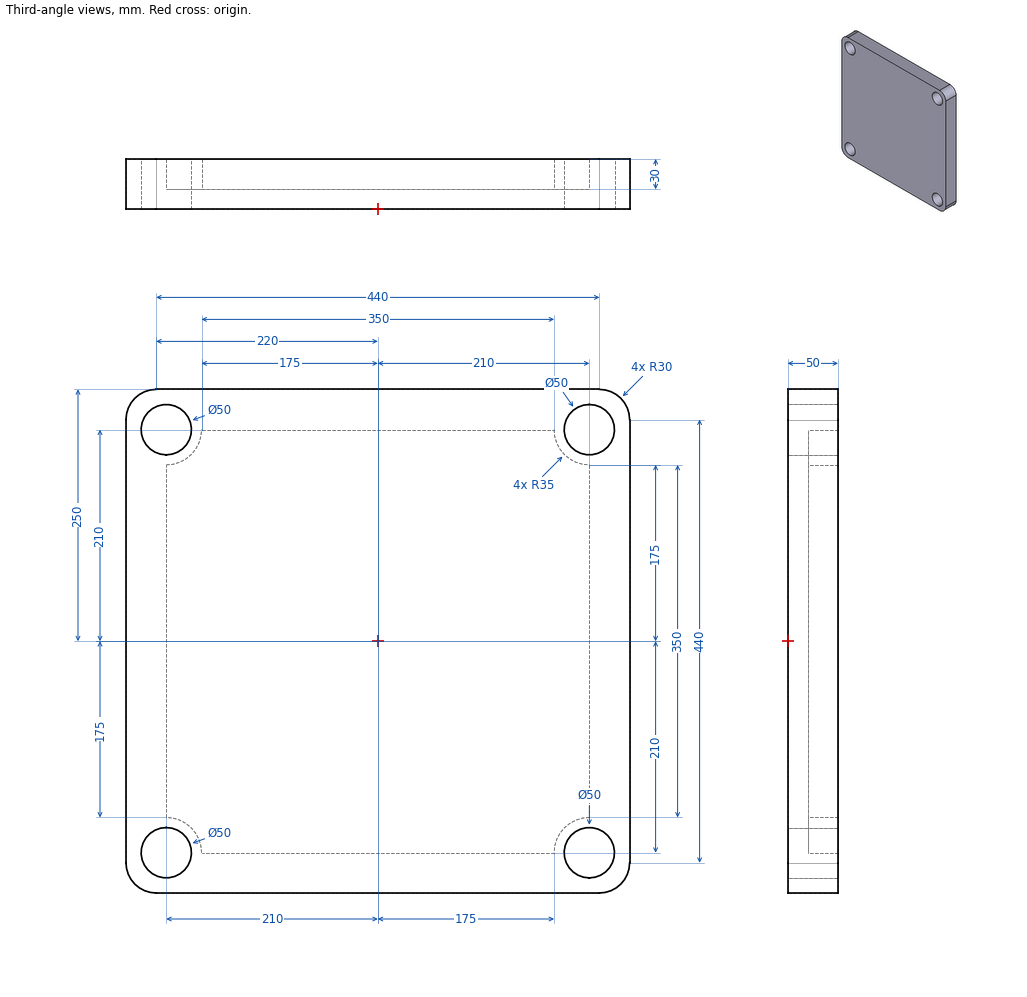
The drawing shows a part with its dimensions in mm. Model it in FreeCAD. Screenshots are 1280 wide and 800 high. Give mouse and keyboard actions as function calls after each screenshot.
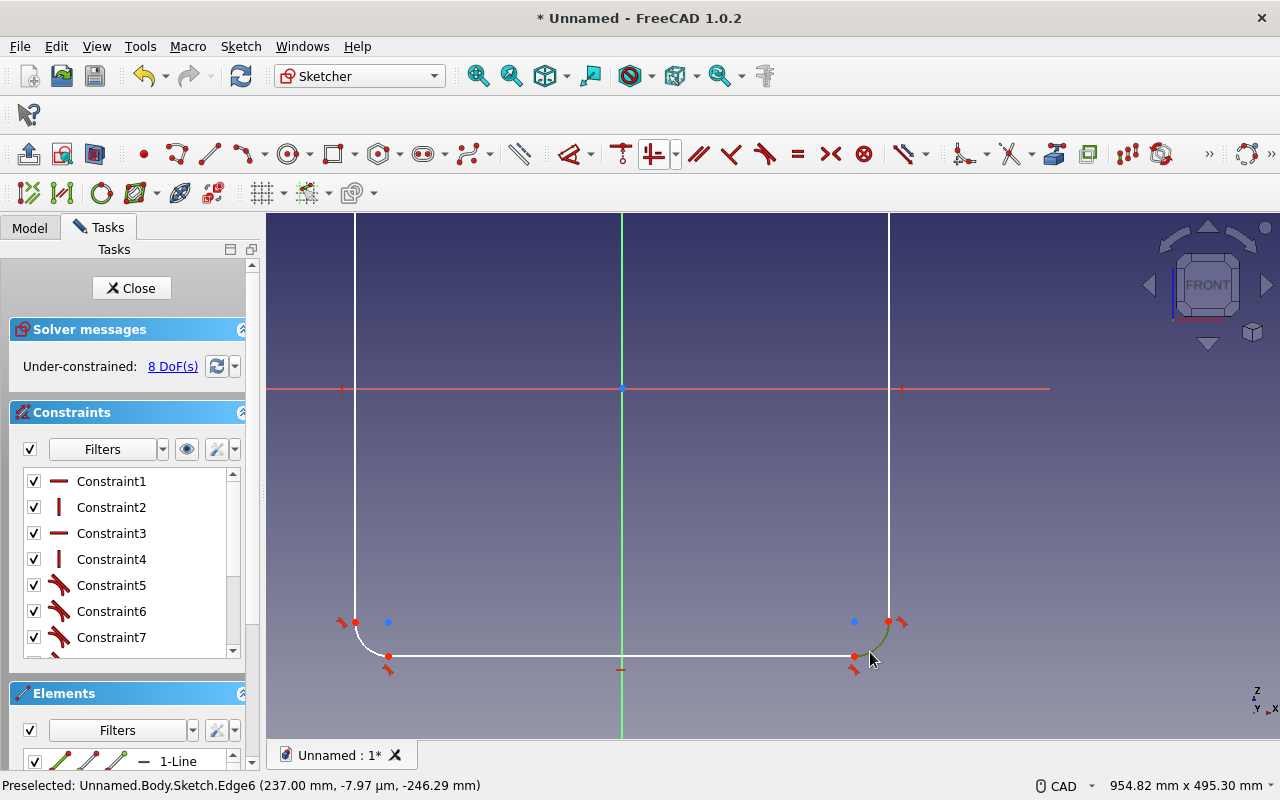
click(359, 638)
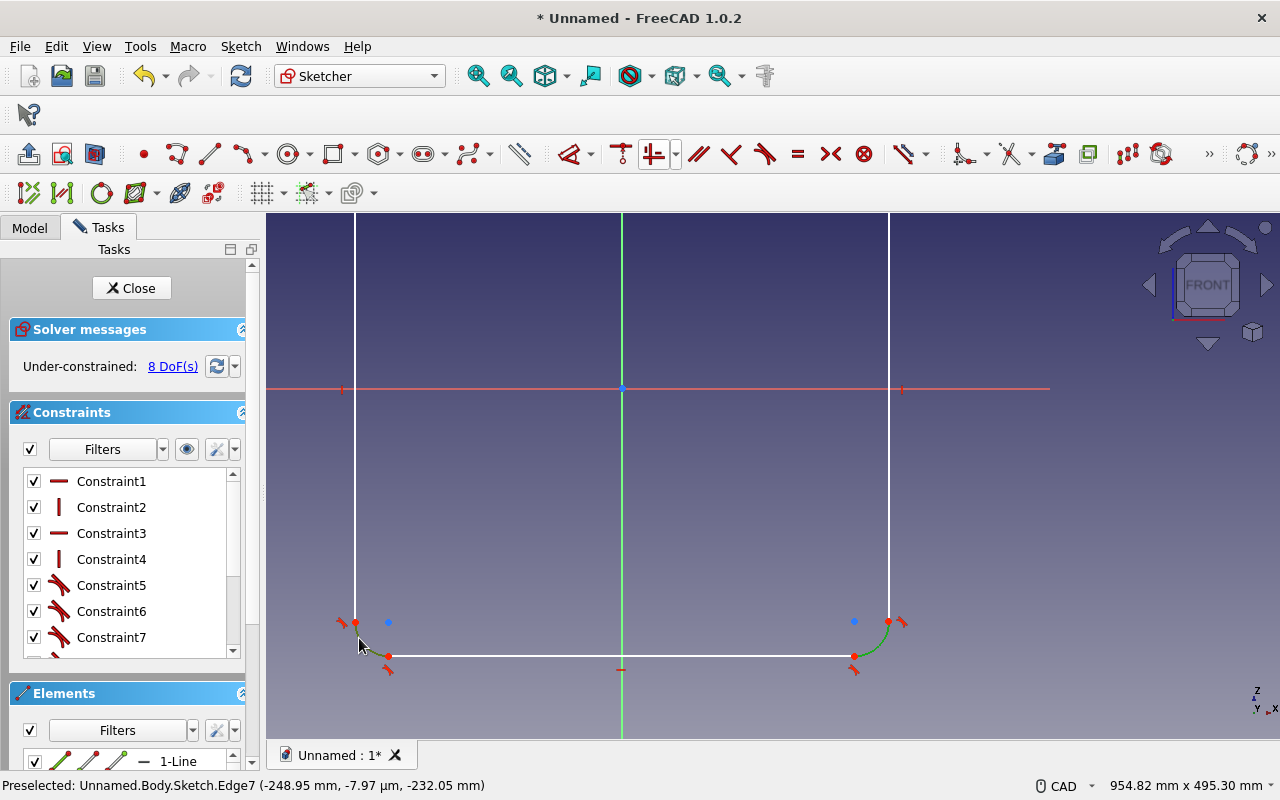
scroll(872, 653, down, 2)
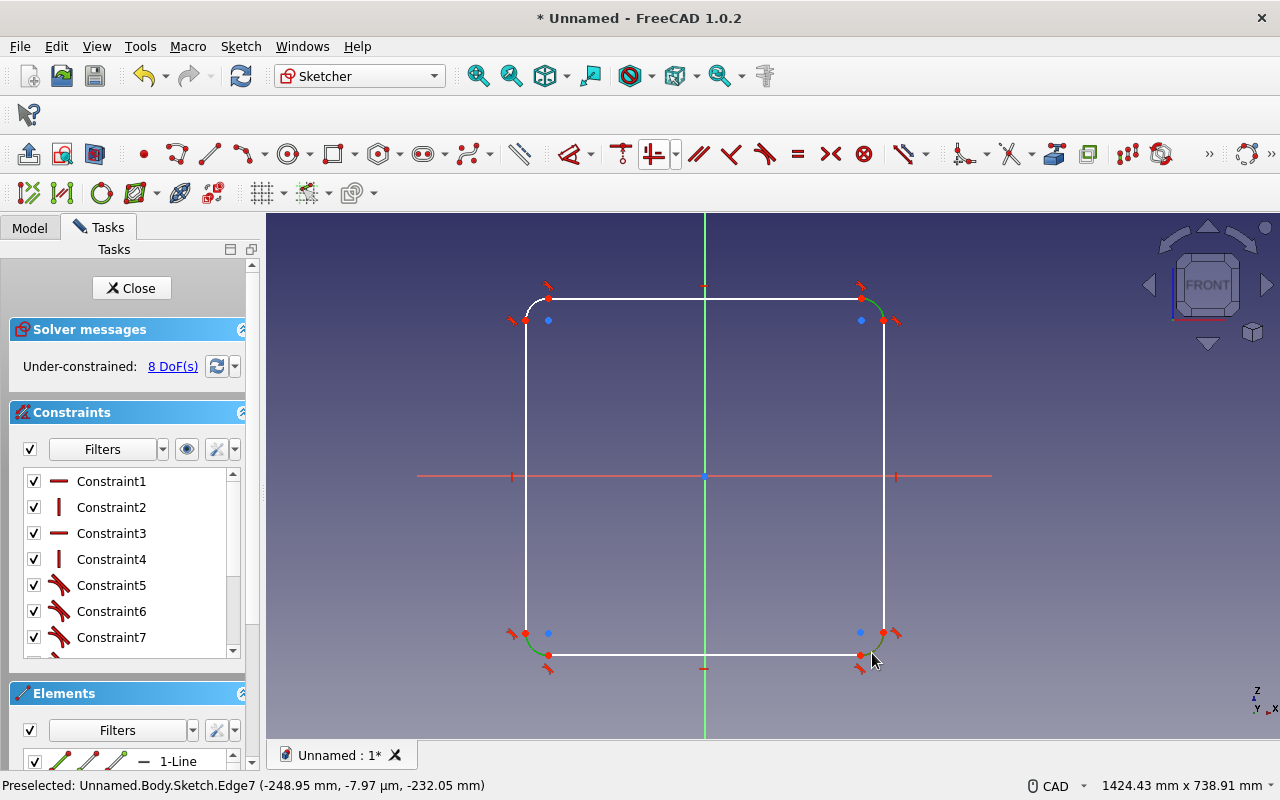
scroll(538, 301, up, 2)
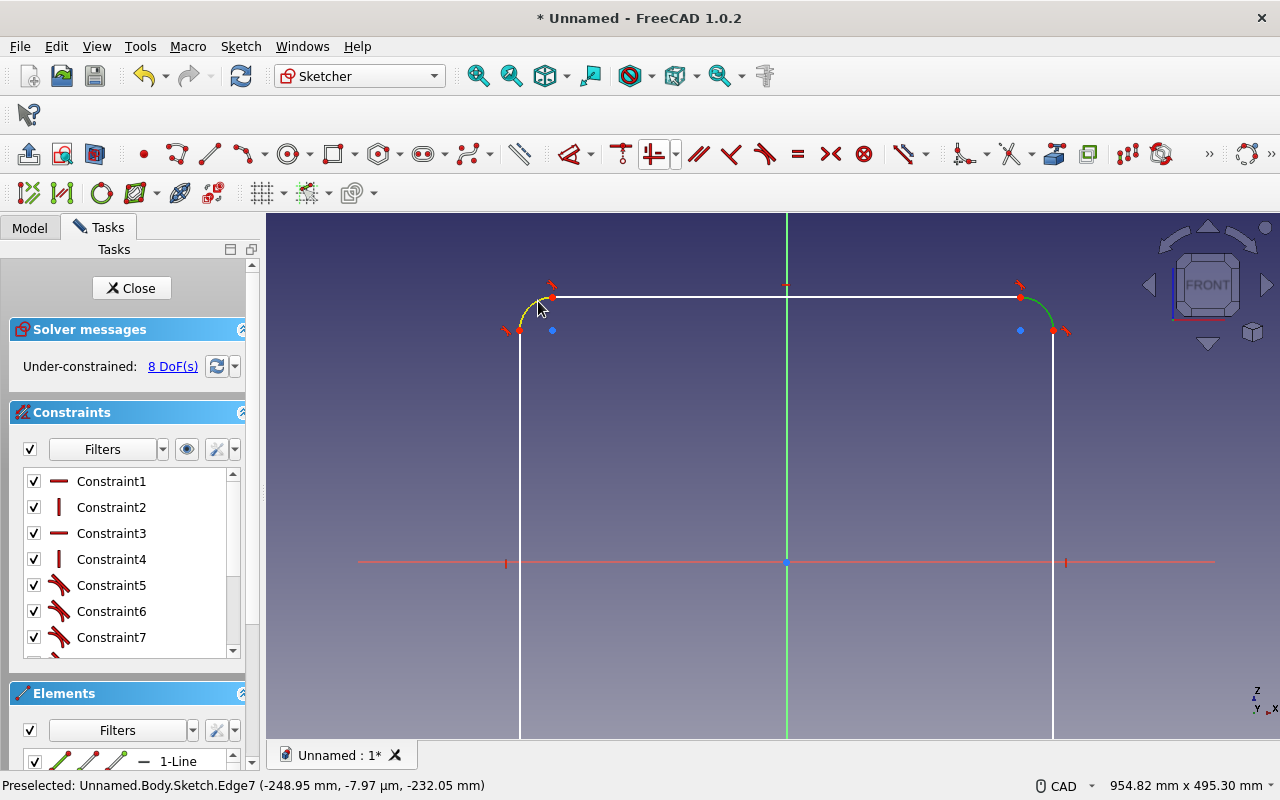
click(538, 301)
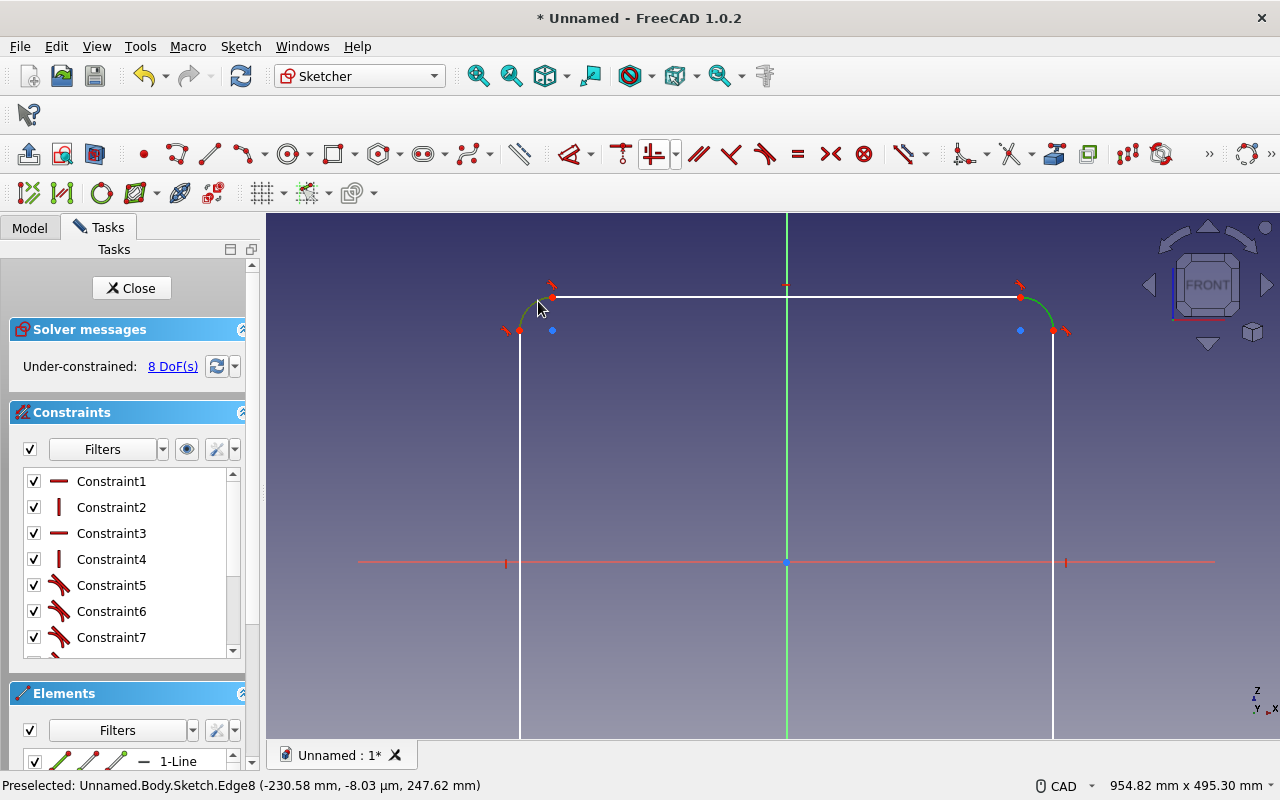
click(798, 154)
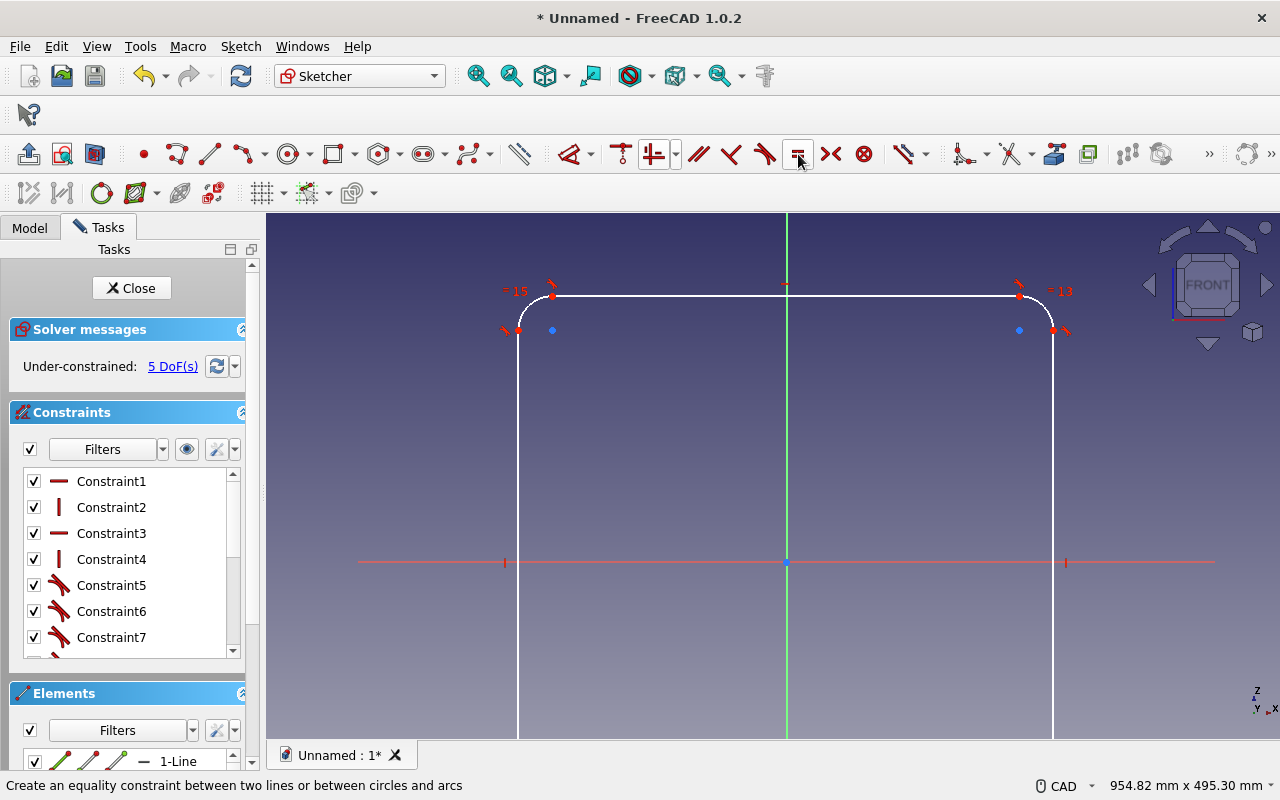
click(568, 154)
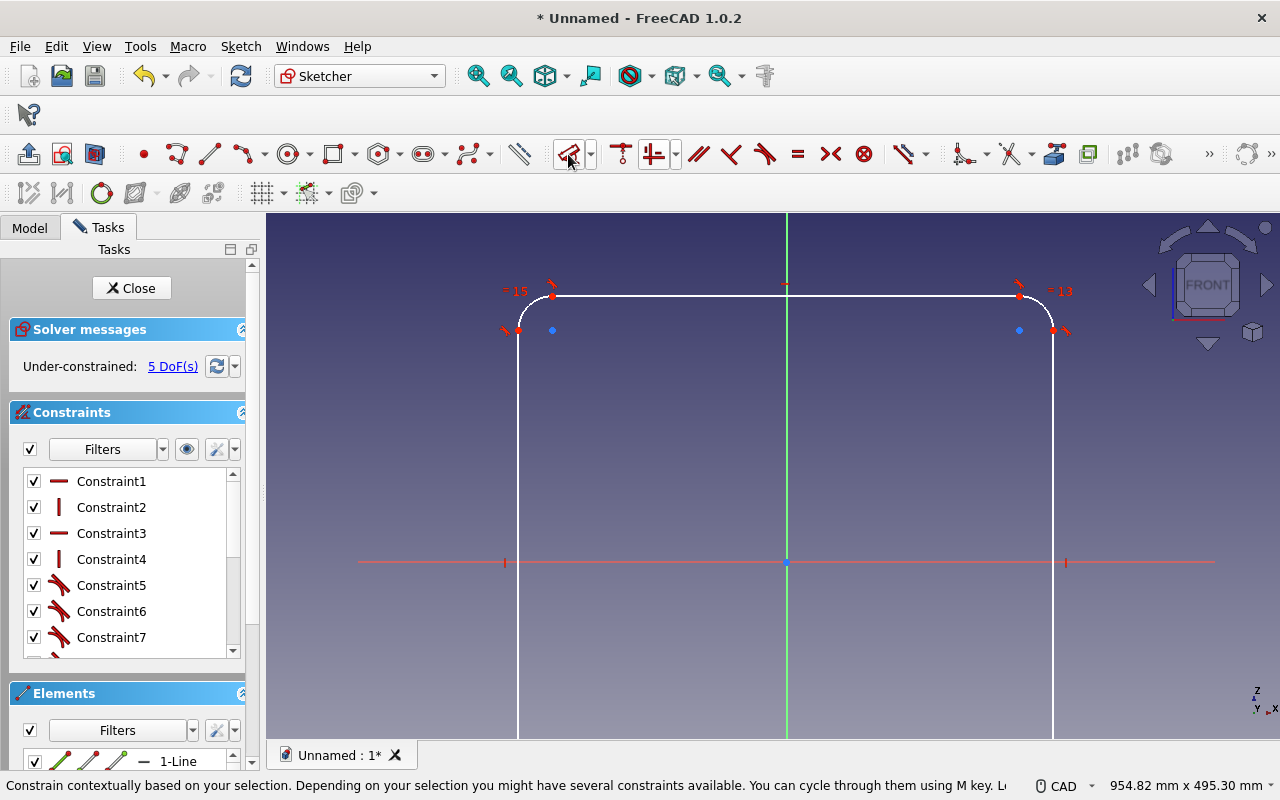
scroll(1050, 315, up, 2)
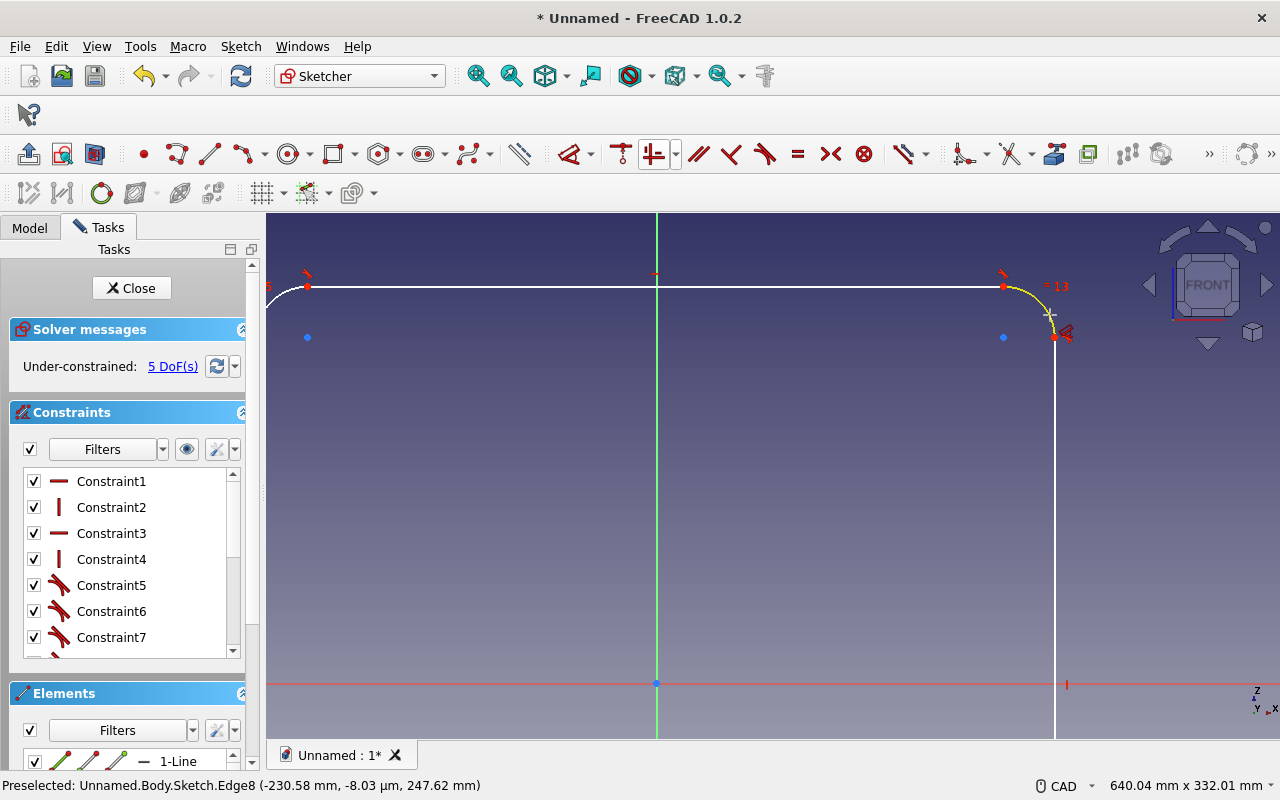
click(1049, 315)
click(1078, 301)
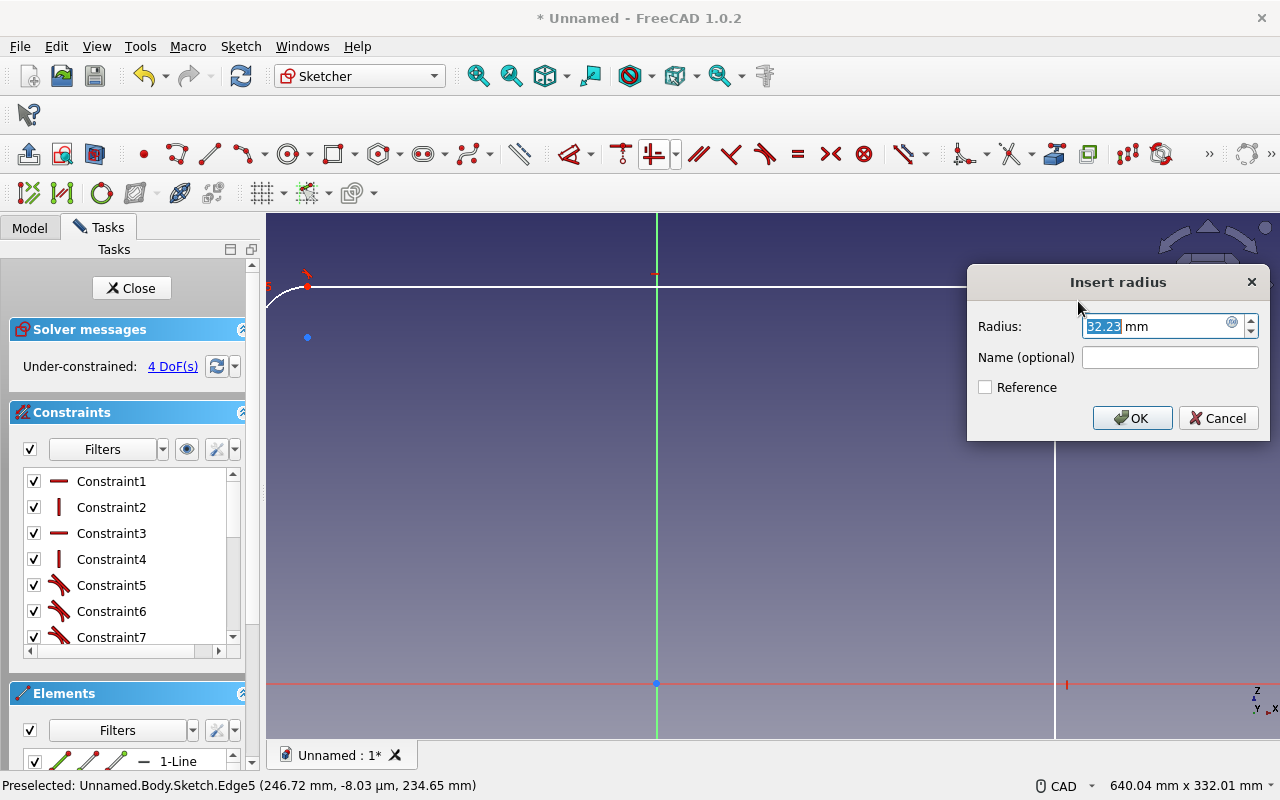
text(30)
key(Return)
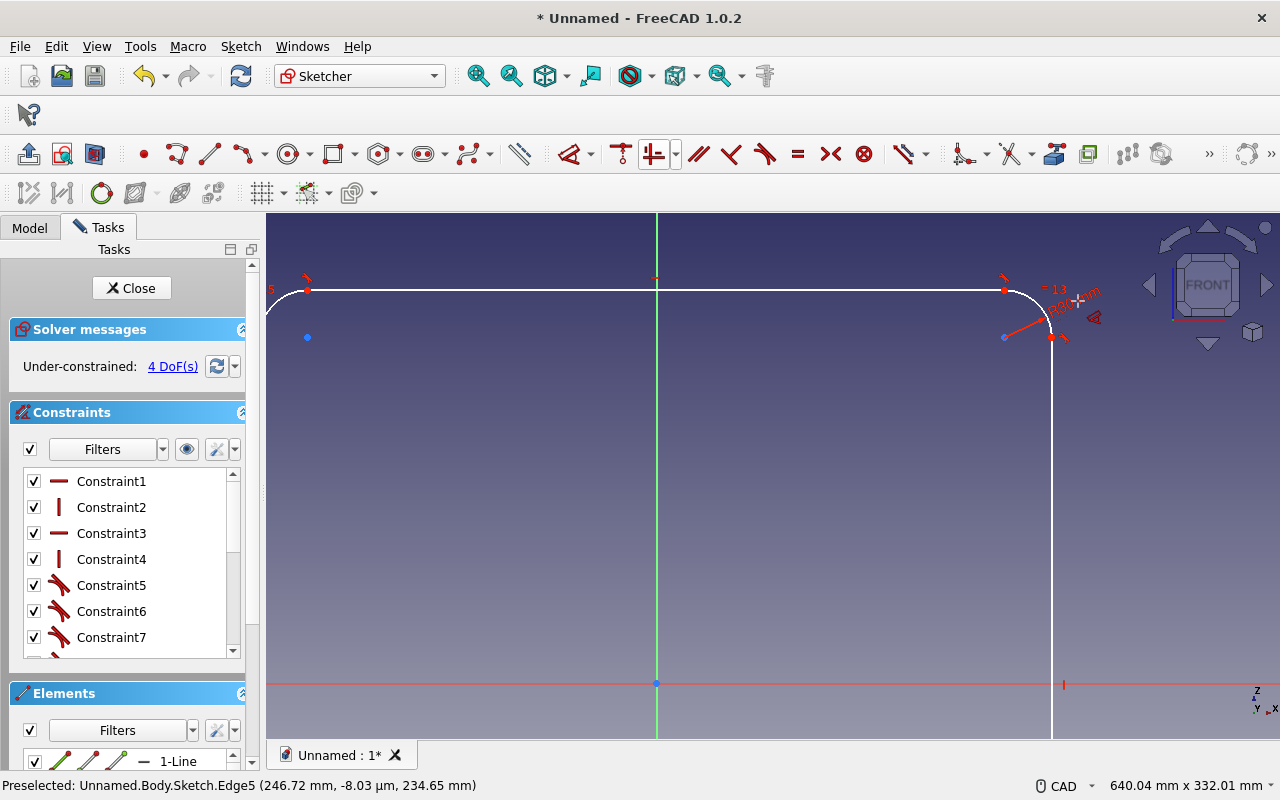
click(517, 290)
click(496, 256)